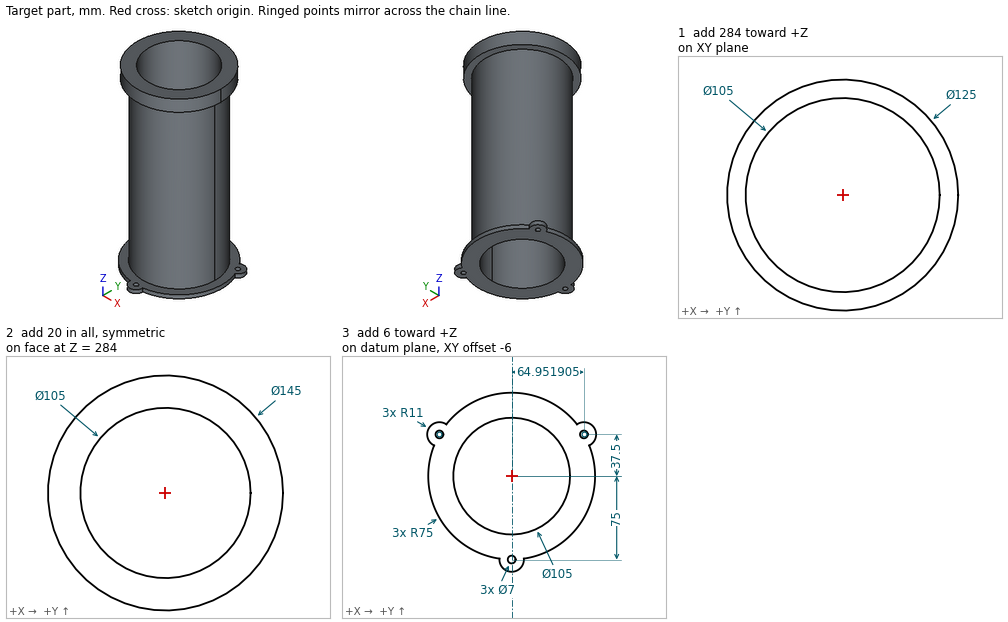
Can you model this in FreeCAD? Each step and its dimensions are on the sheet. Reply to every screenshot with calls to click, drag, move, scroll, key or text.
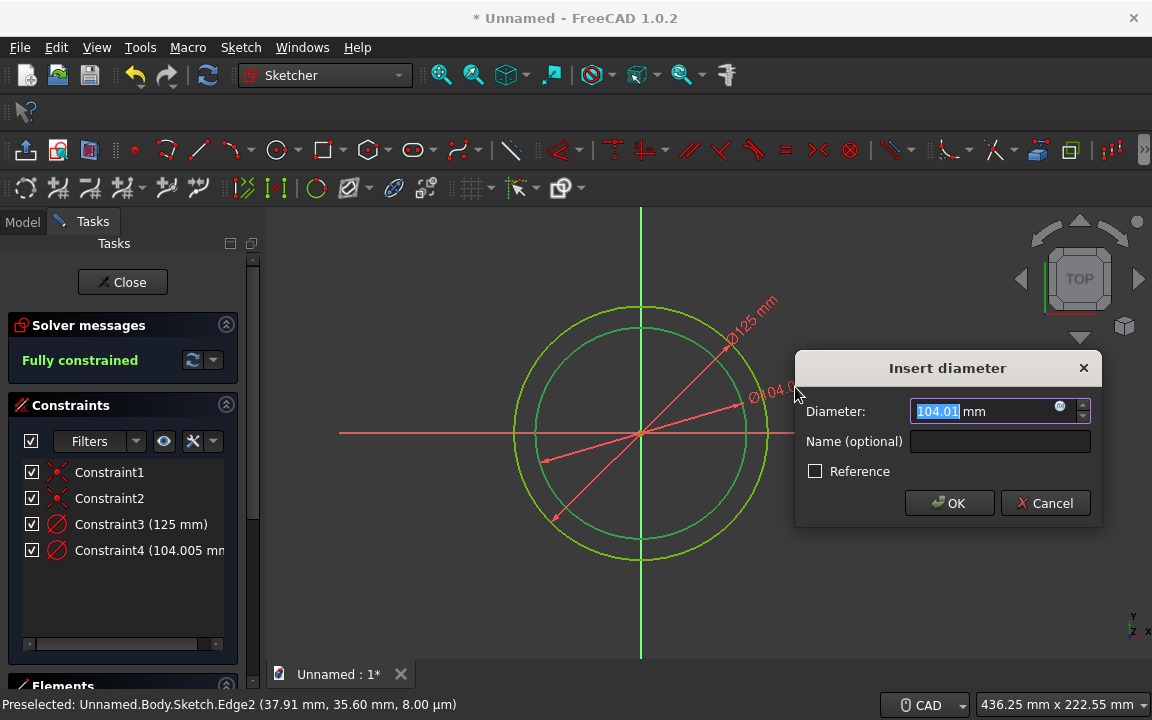
text(105)
key(Return)
key(Escape)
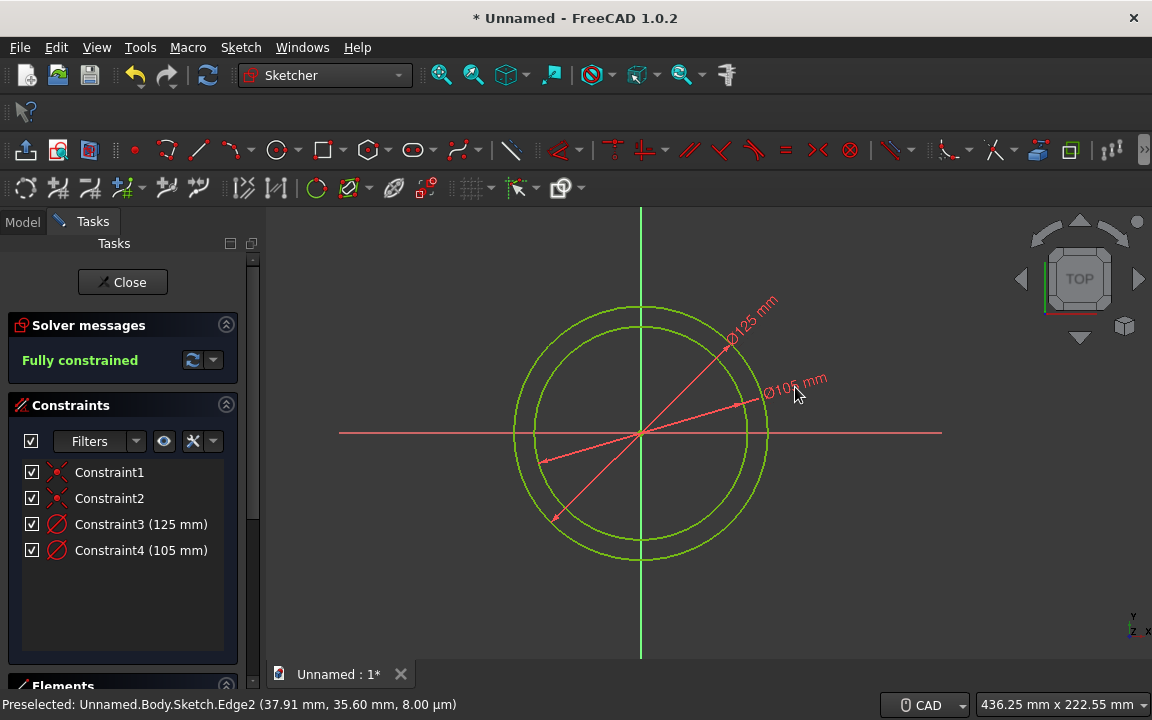
click(123, 282)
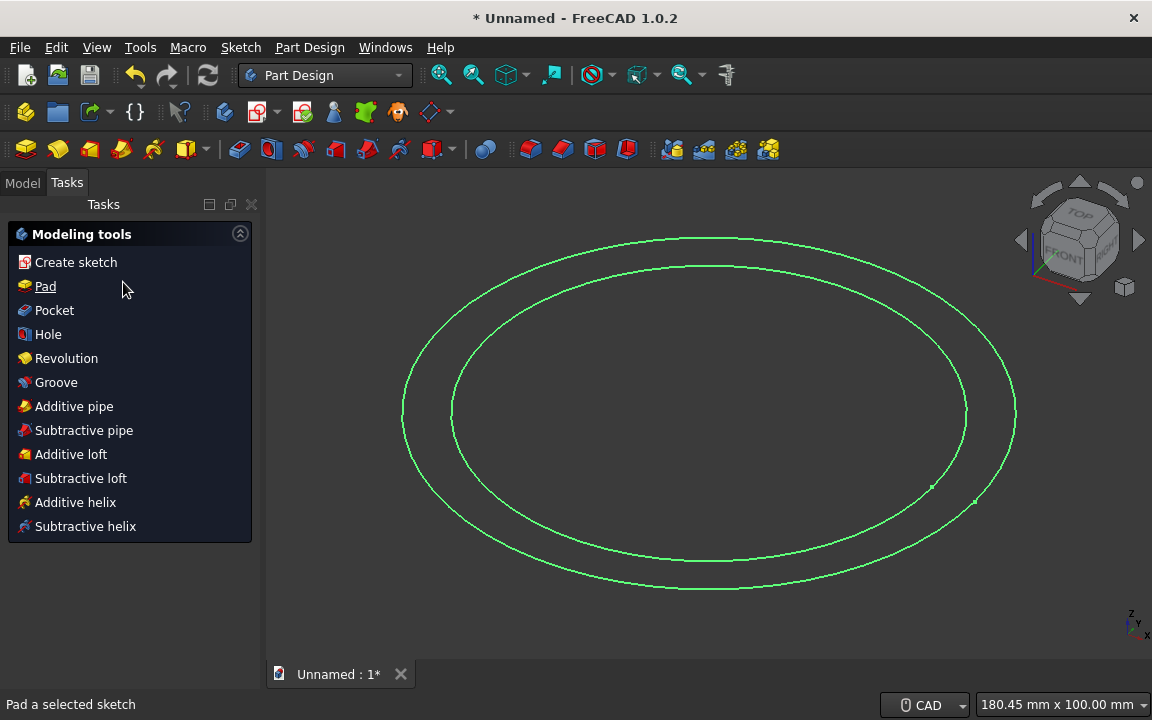
click(26, 150)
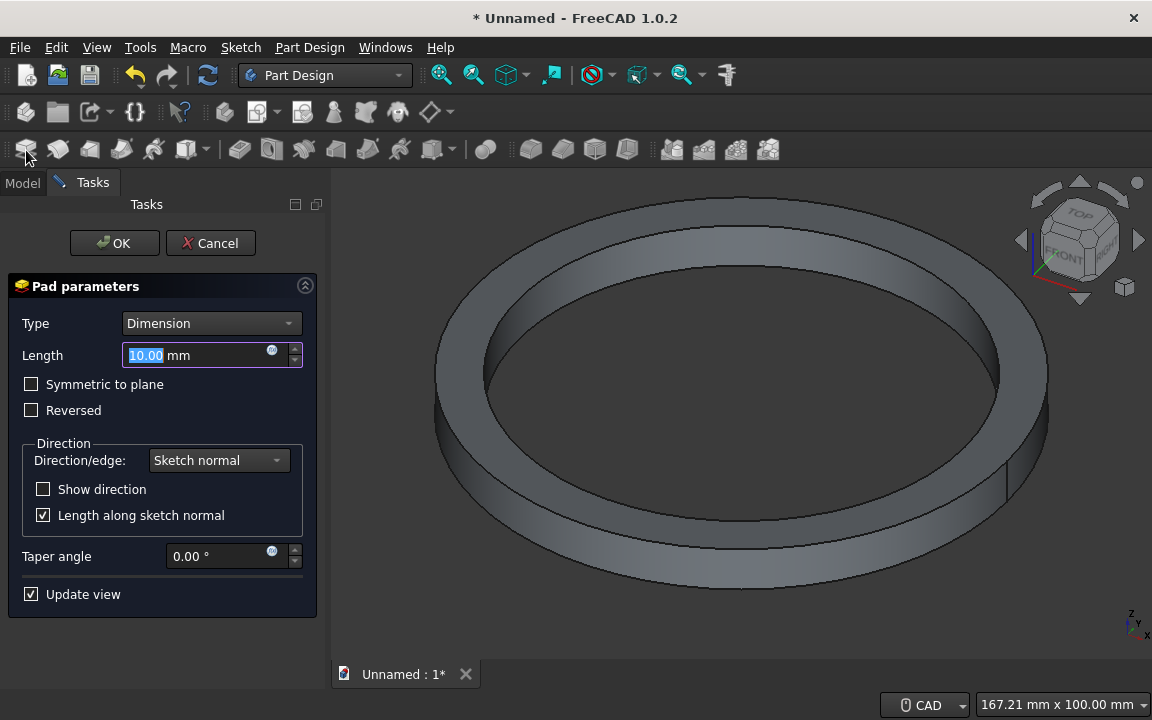
text(284)
key(Tab)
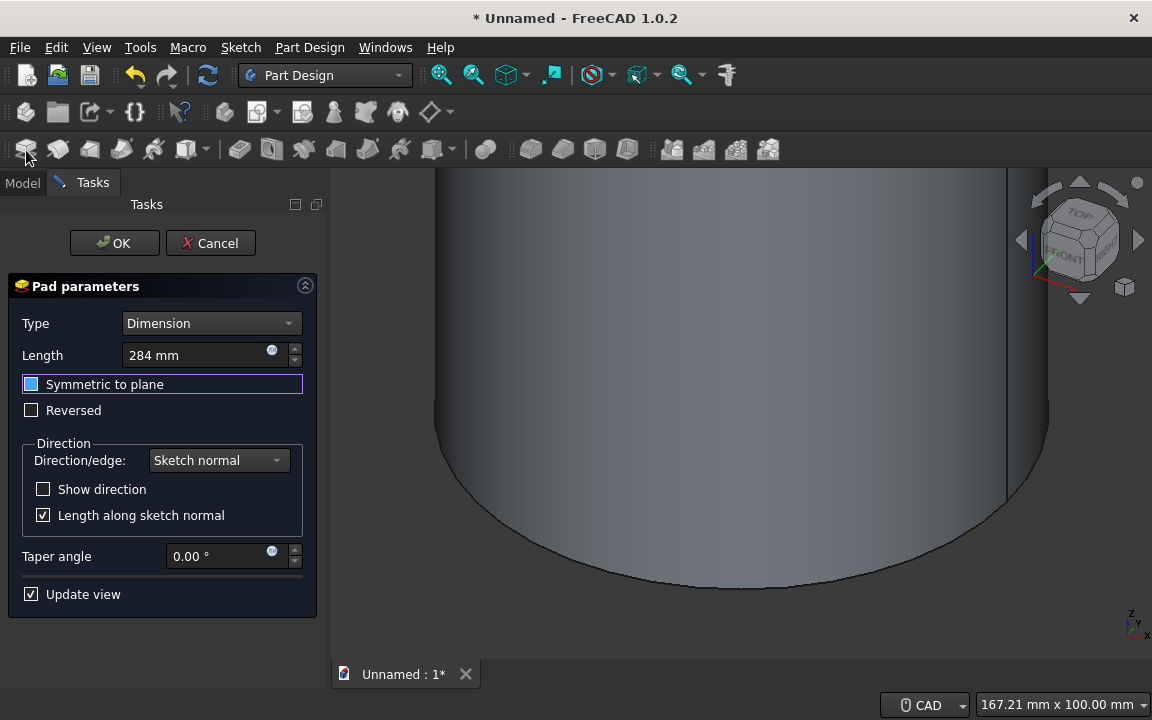
click(115, 243)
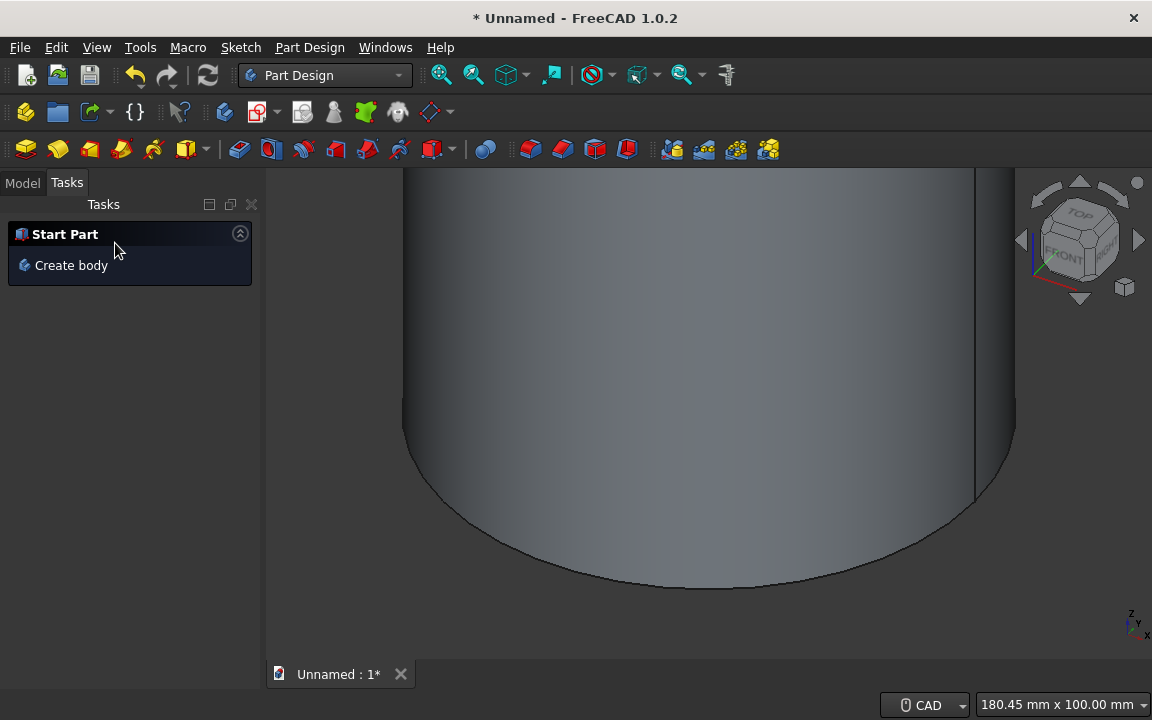
click(442, 76)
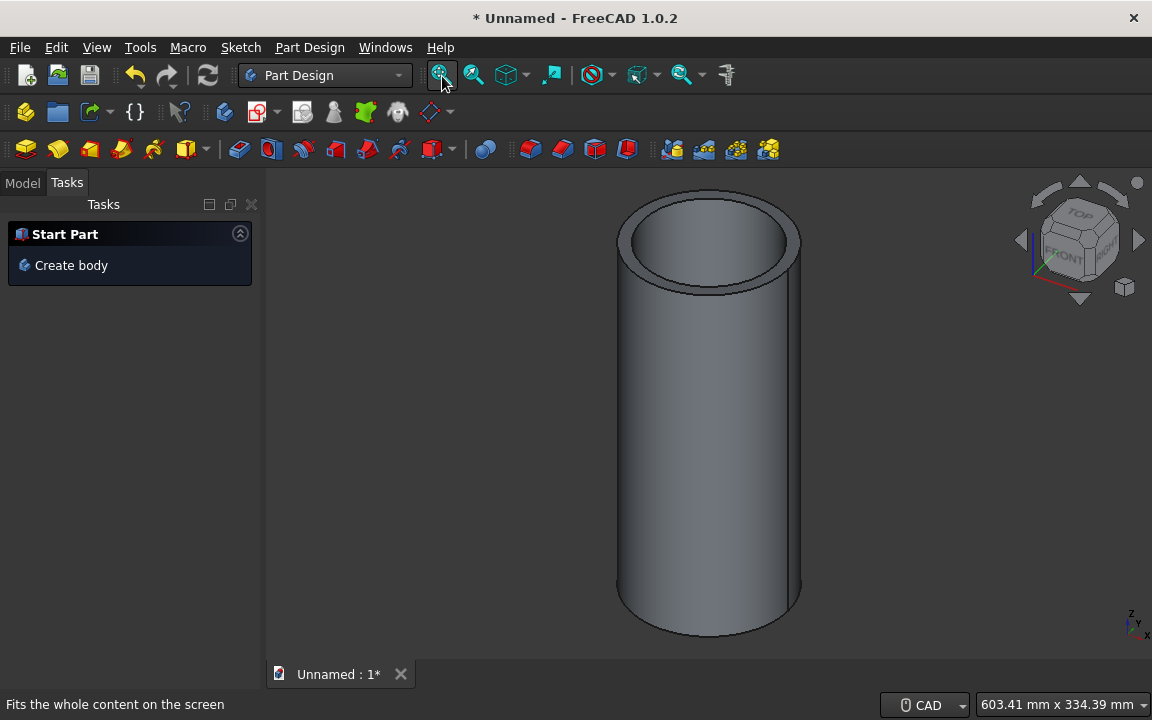
scroll(654, 206, up, 4)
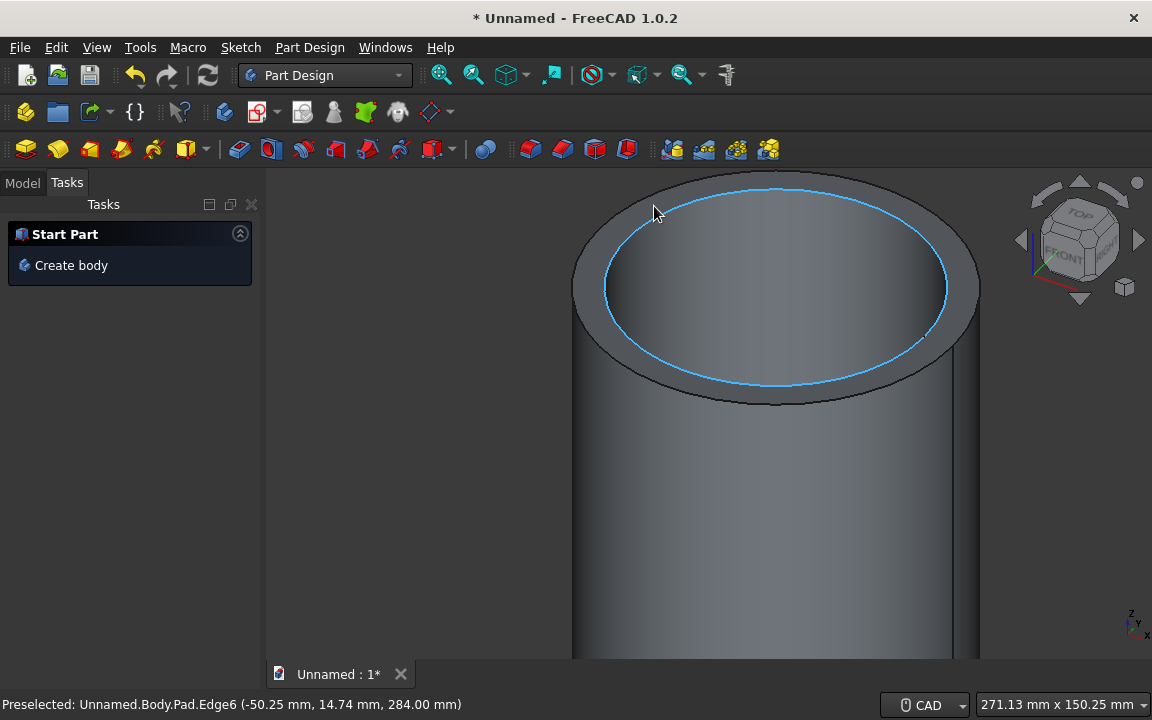
click(653, 207)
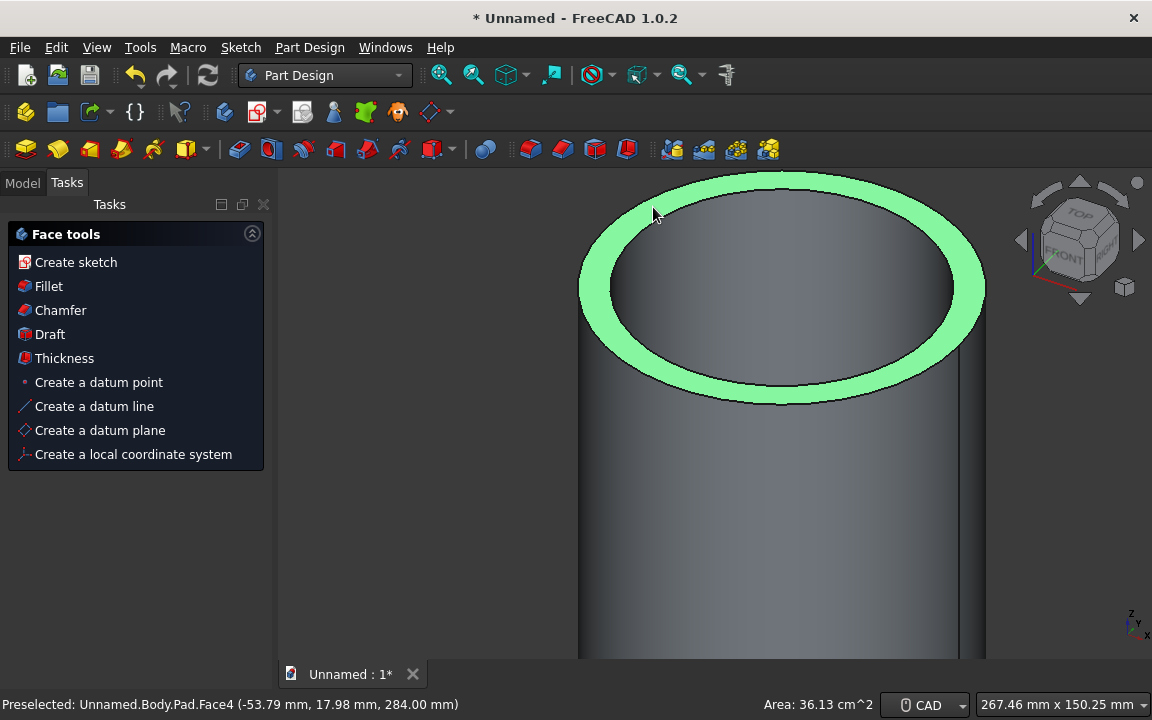
click(258, 112)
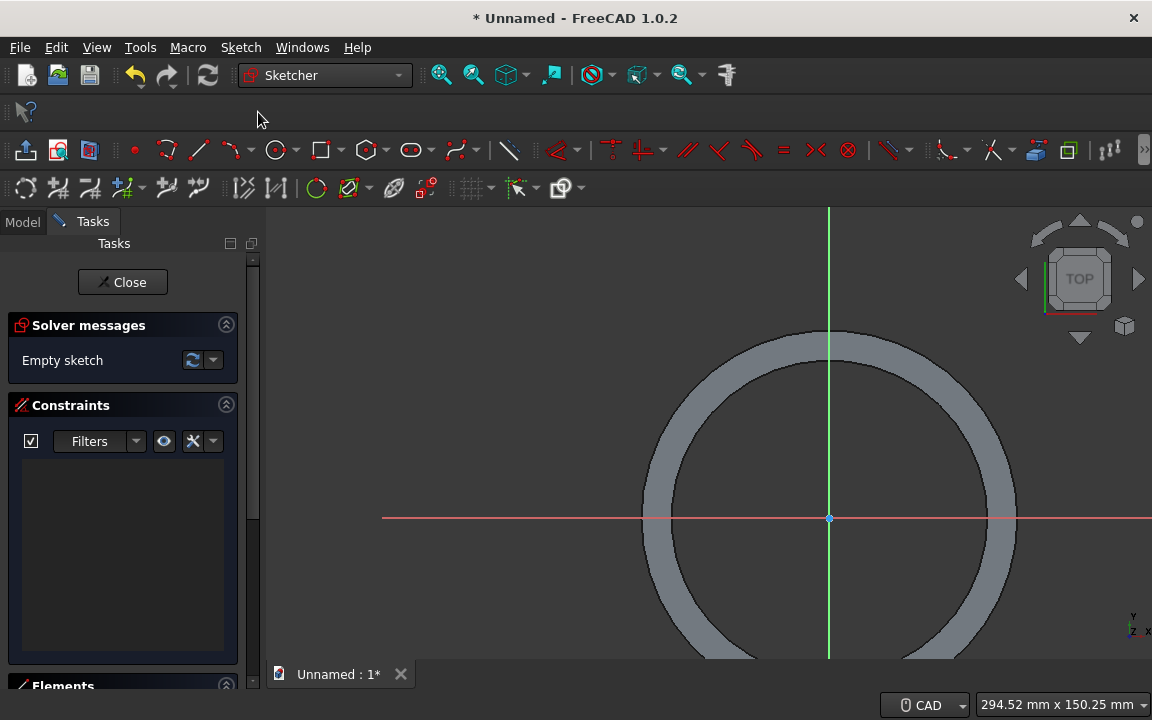
scroll(294, 259, down, 2)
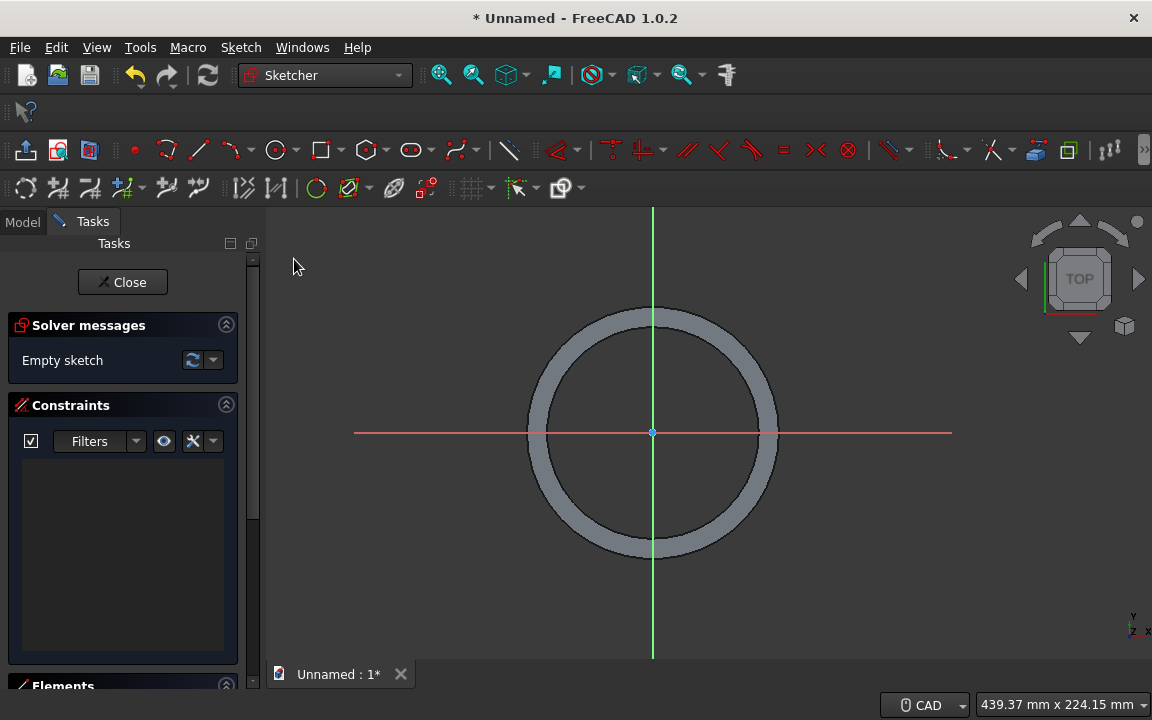
click(276, 150)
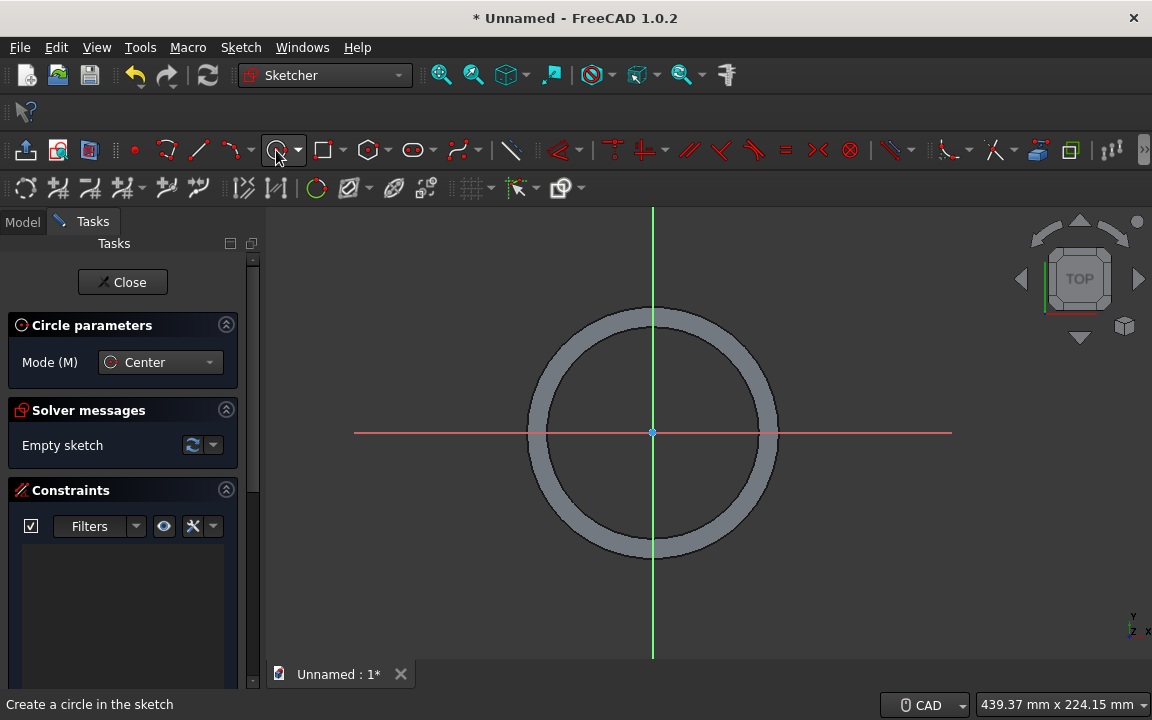
click(653, 433)
click(756, 330)